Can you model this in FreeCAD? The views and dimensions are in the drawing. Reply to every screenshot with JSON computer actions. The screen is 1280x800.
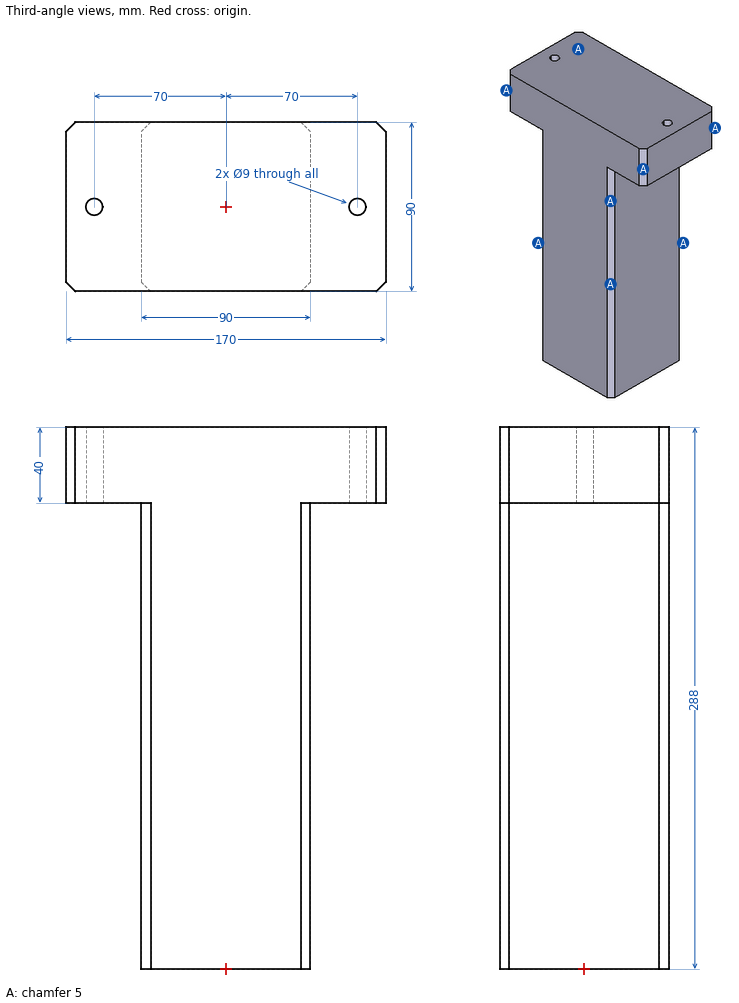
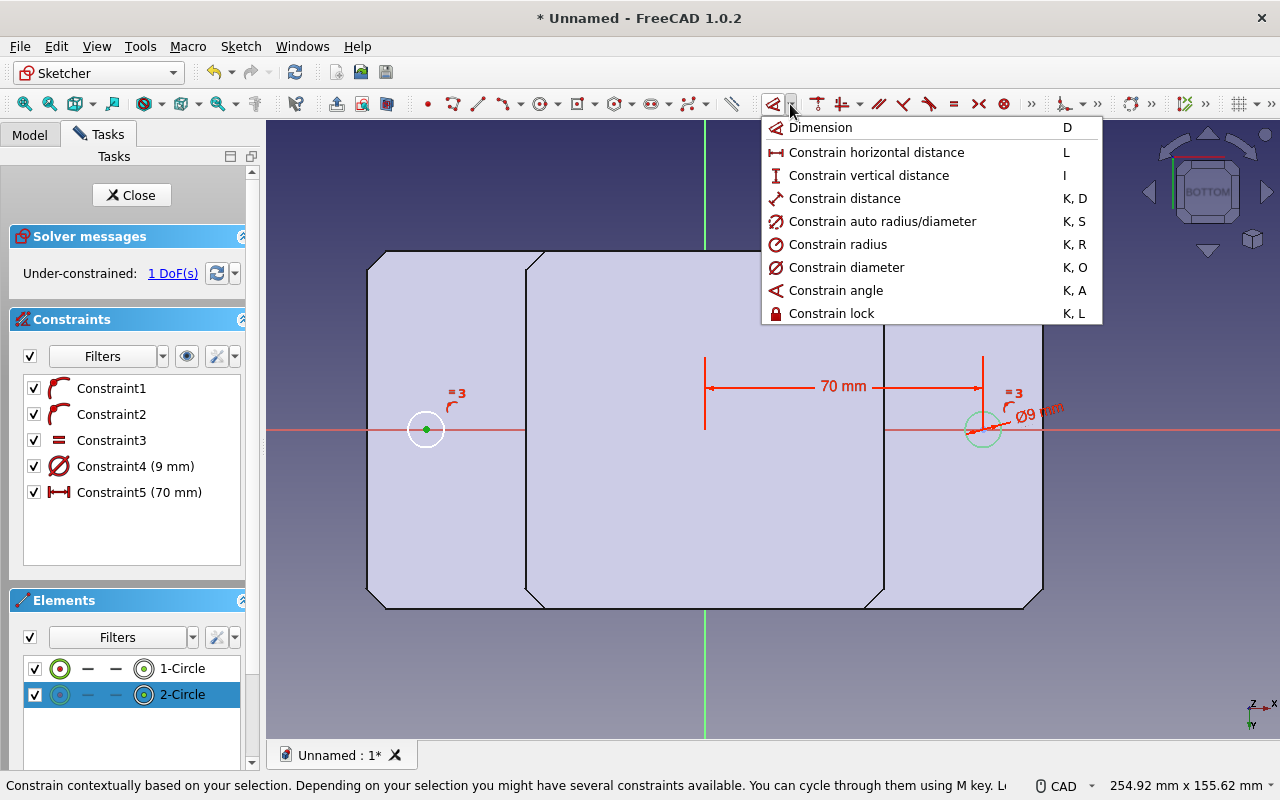
{"action": "left_click", "coordinate": [932, 152]}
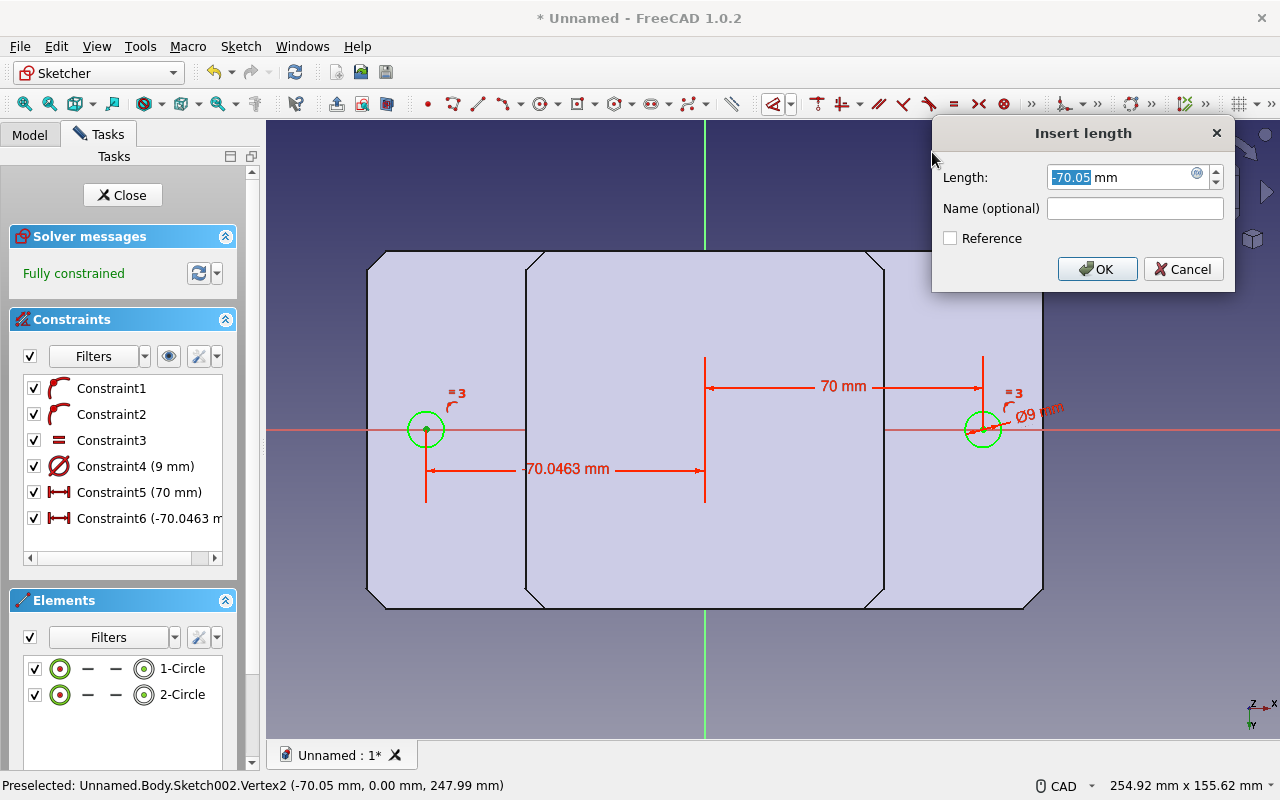
{"action": "type", "text": "-70"}
{"action": "key", "text": "Return"}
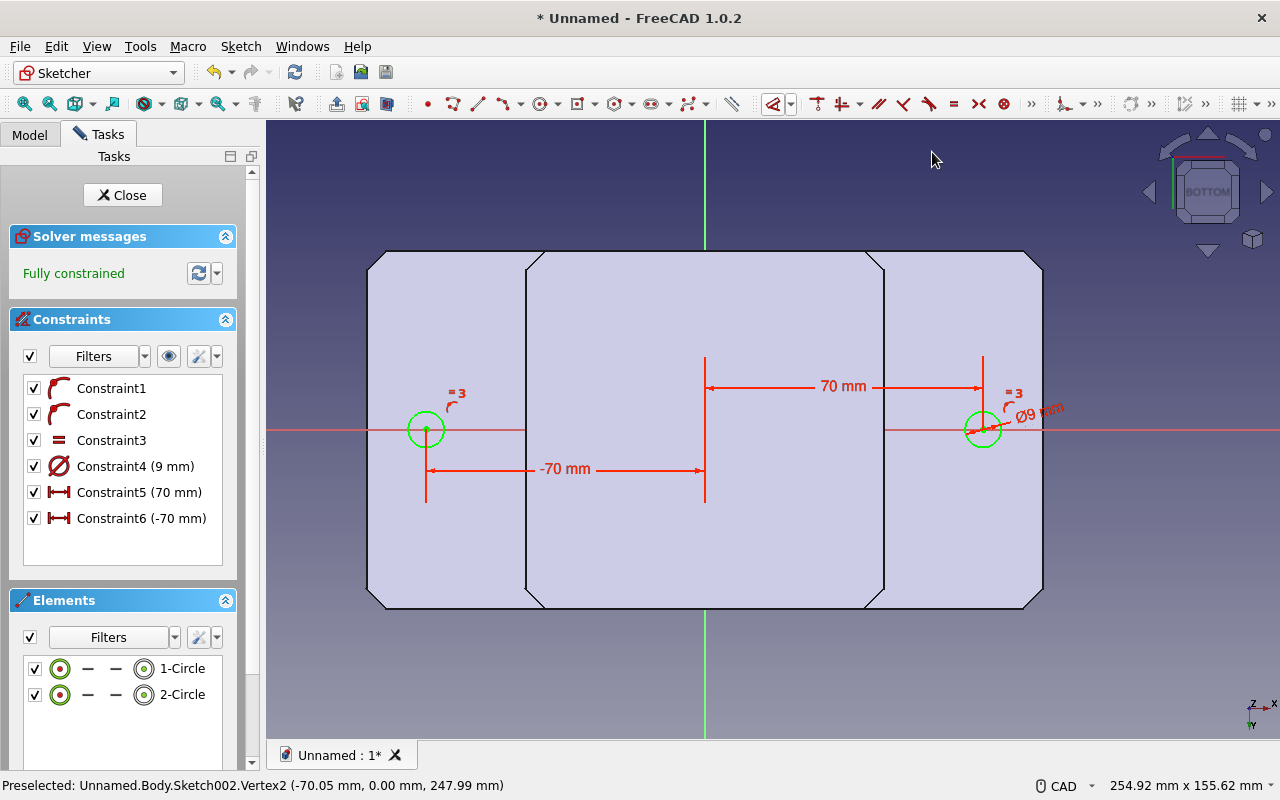
{"action": "left_click", "coordinate": [123, 195]}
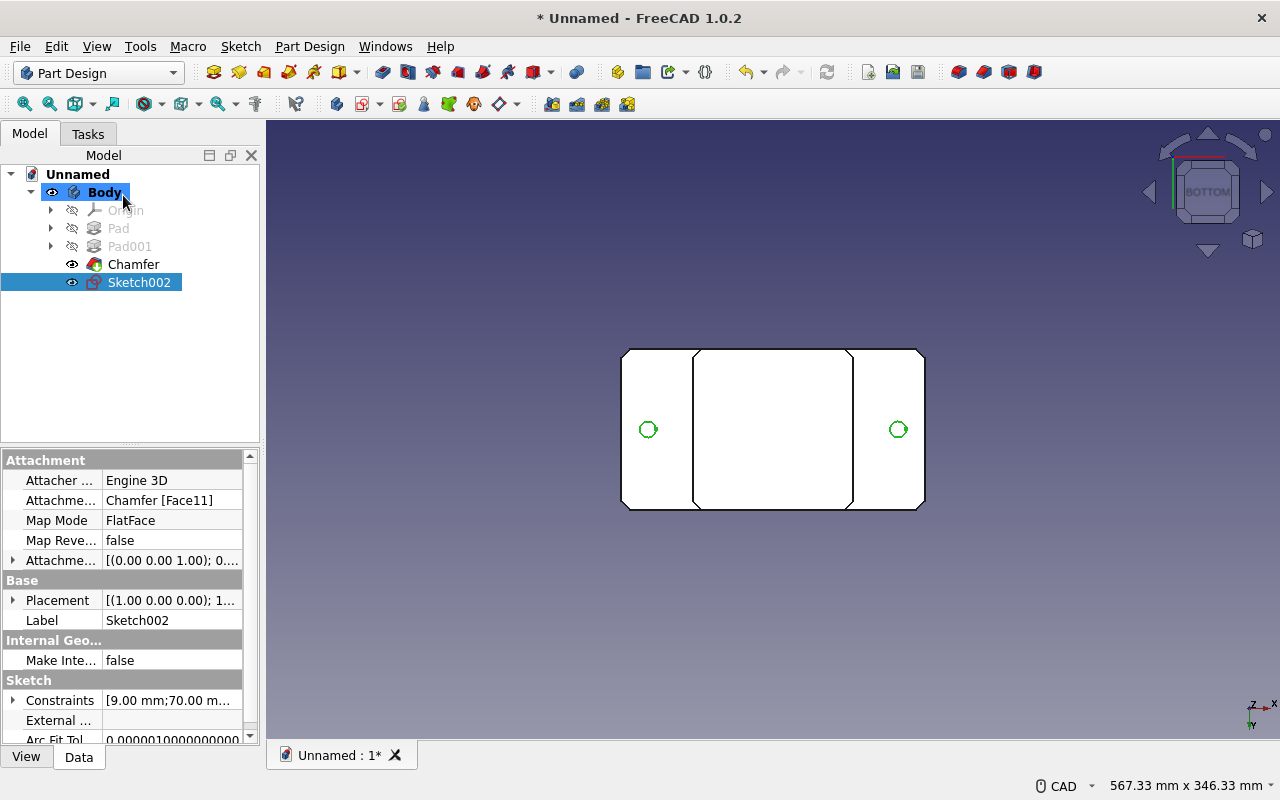
{"action": "left_click", "coordinate": [408, 72]}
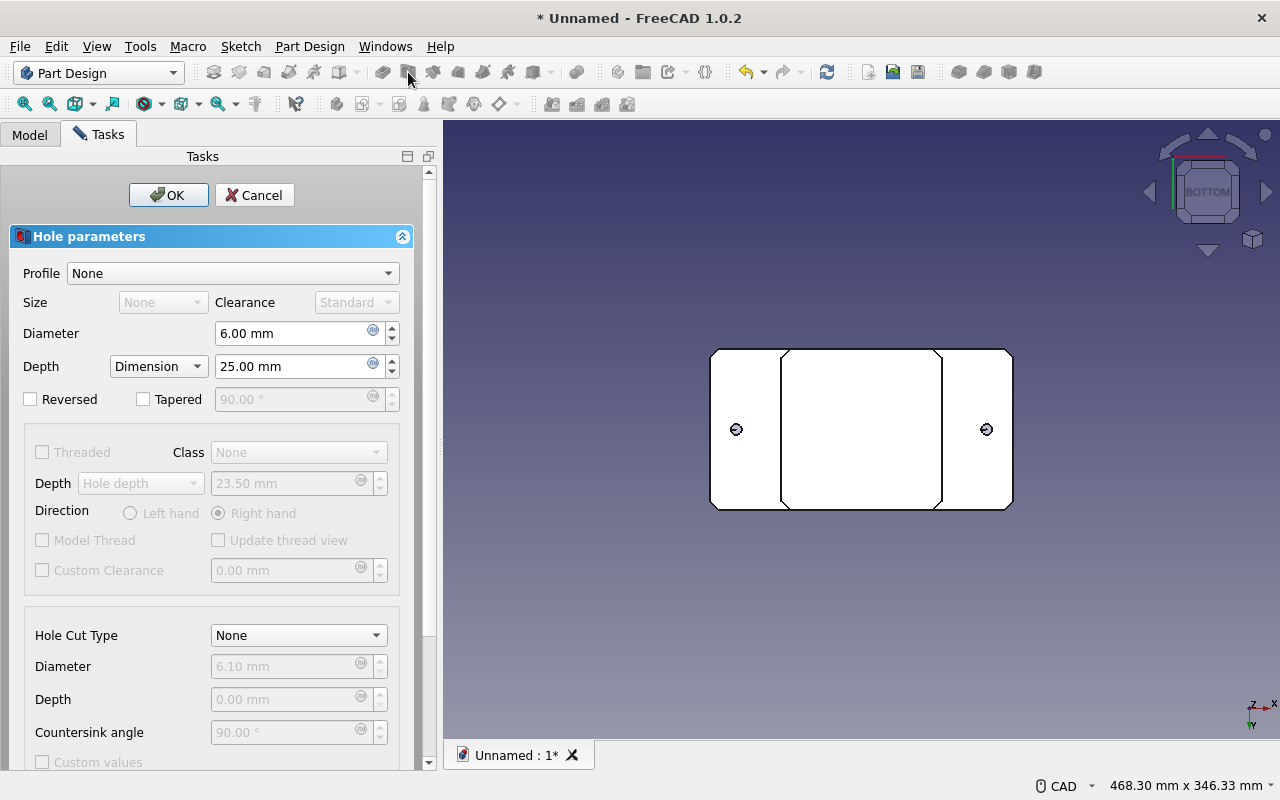
{"action": "triple_click", "coordinate": [300, 334]}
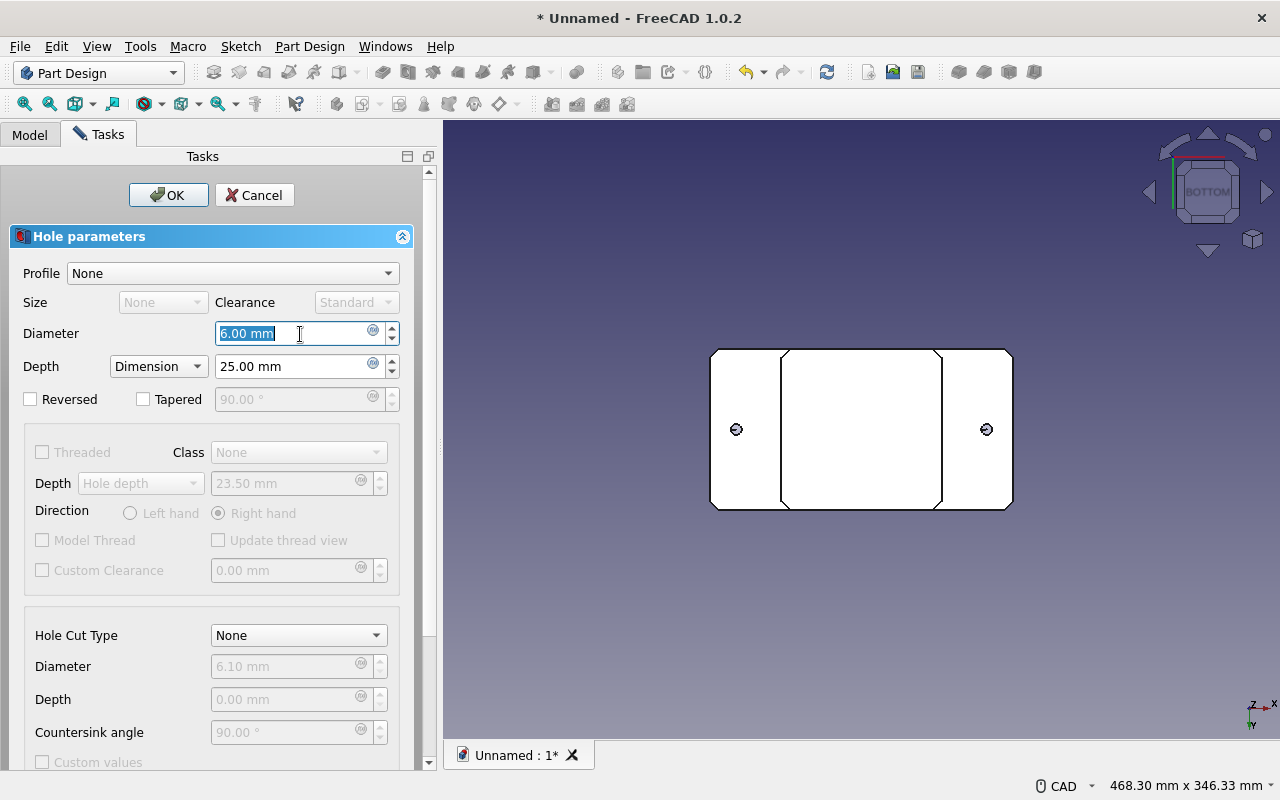
{"action": "type", "text": "9"}
{"action": "key", "text": "Tab"}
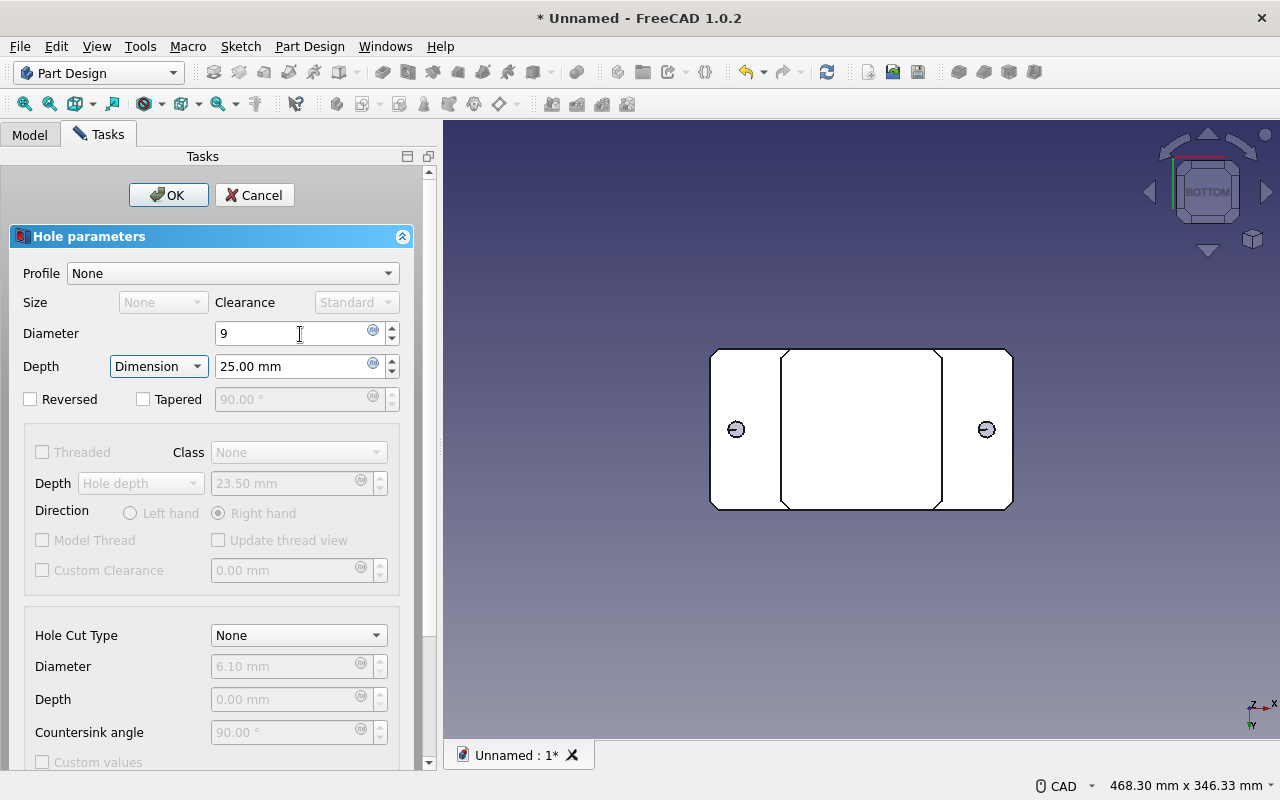
{"action": "left_click", "coordinate": [160, 366]}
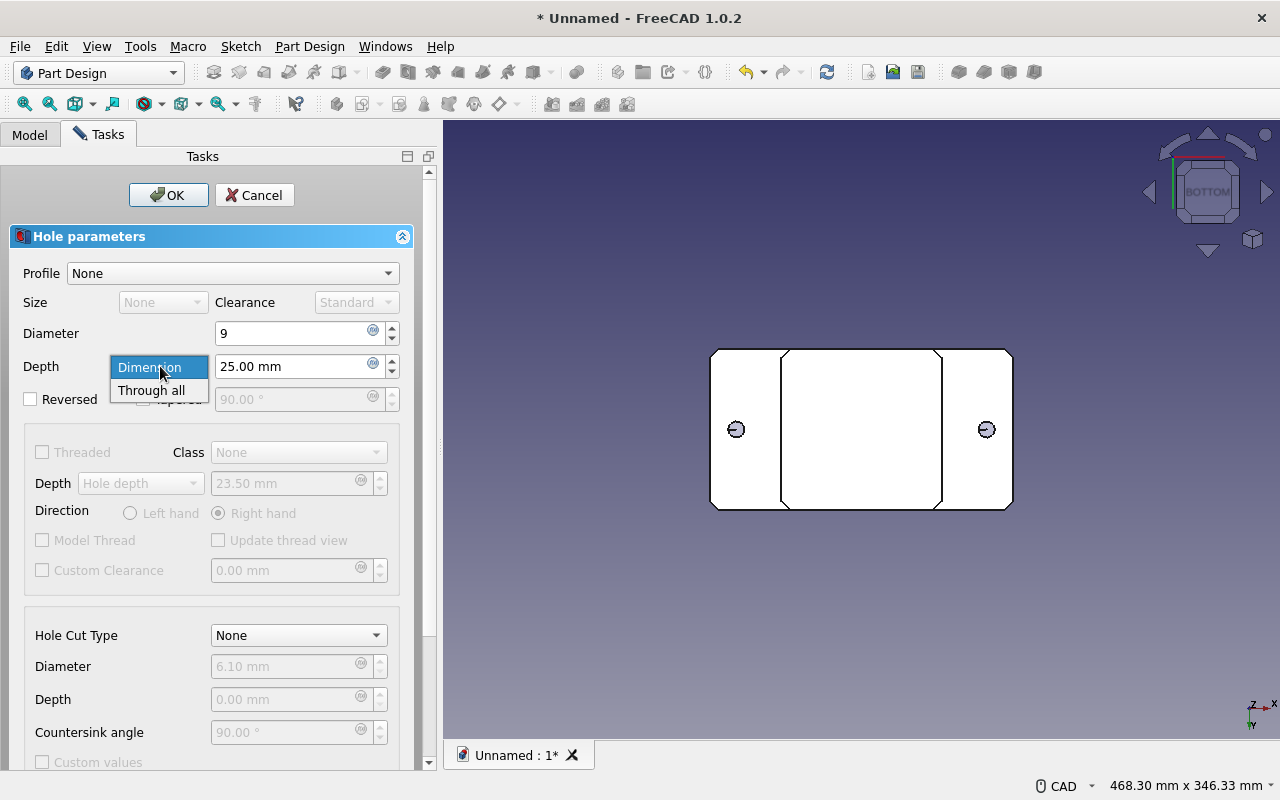
{"action": "left_click", "coordinate": [158, 390]}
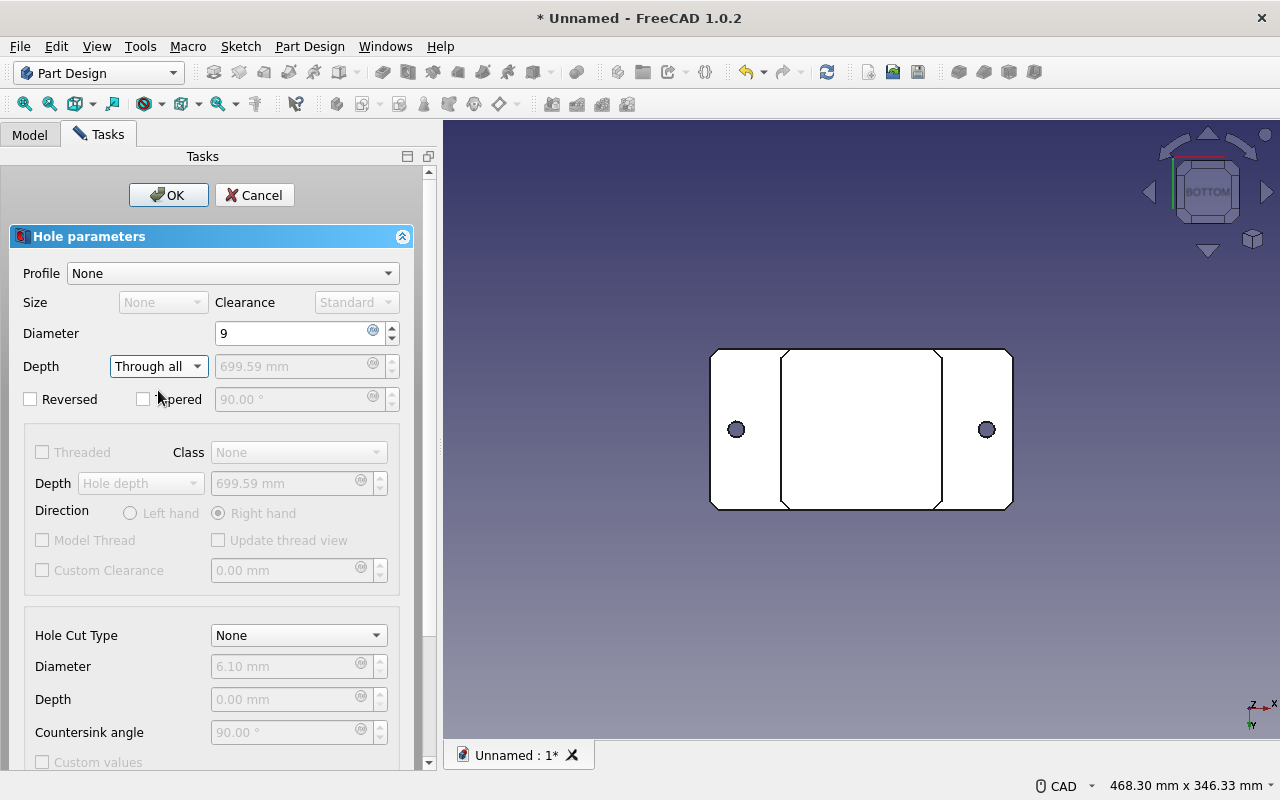
{"action": "left_click", "coordinate": [169, 195]}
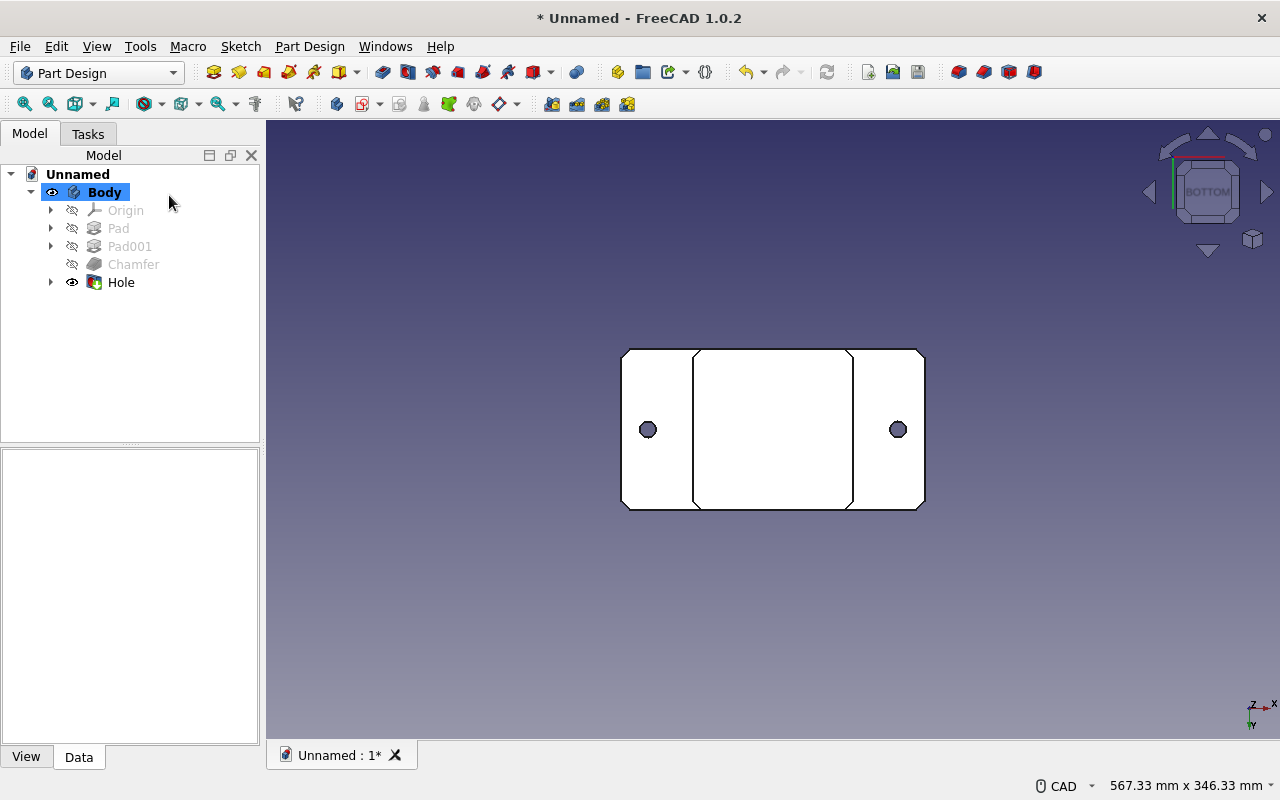
{"action": "key", "text": "0"}